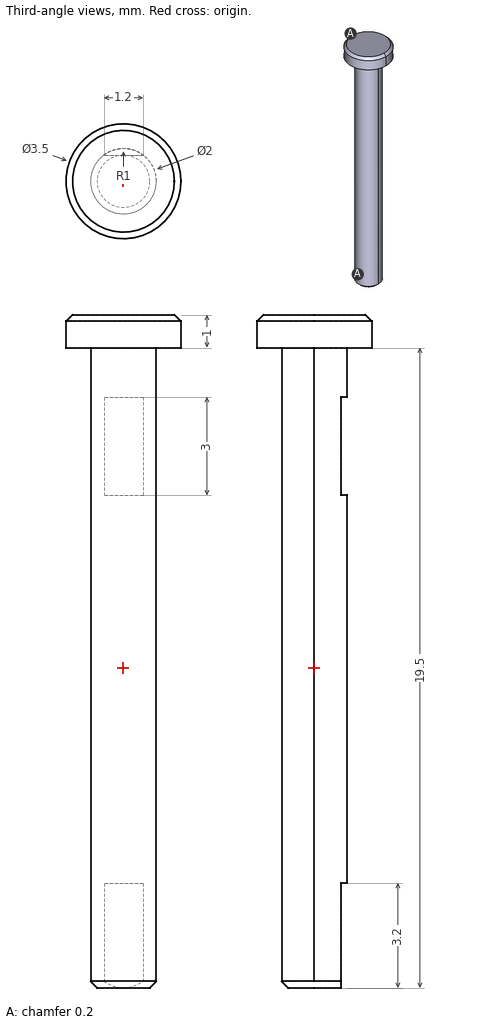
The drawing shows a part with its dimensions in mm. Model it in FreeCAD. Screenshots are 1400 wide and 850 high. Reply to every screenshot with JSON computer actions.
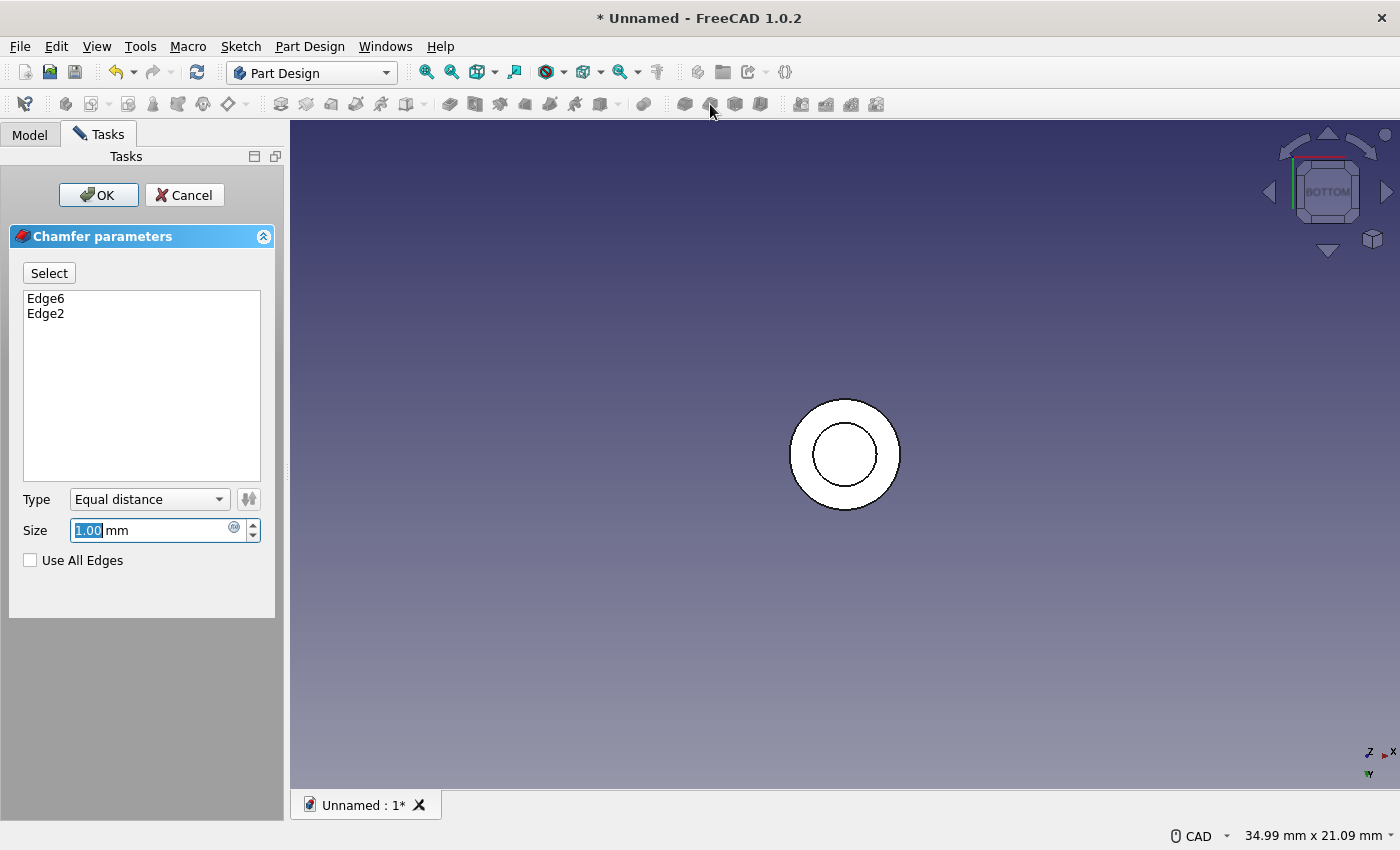
{"action": "type", "text": "0.2"}
{"action": "key", "text": "Tab"}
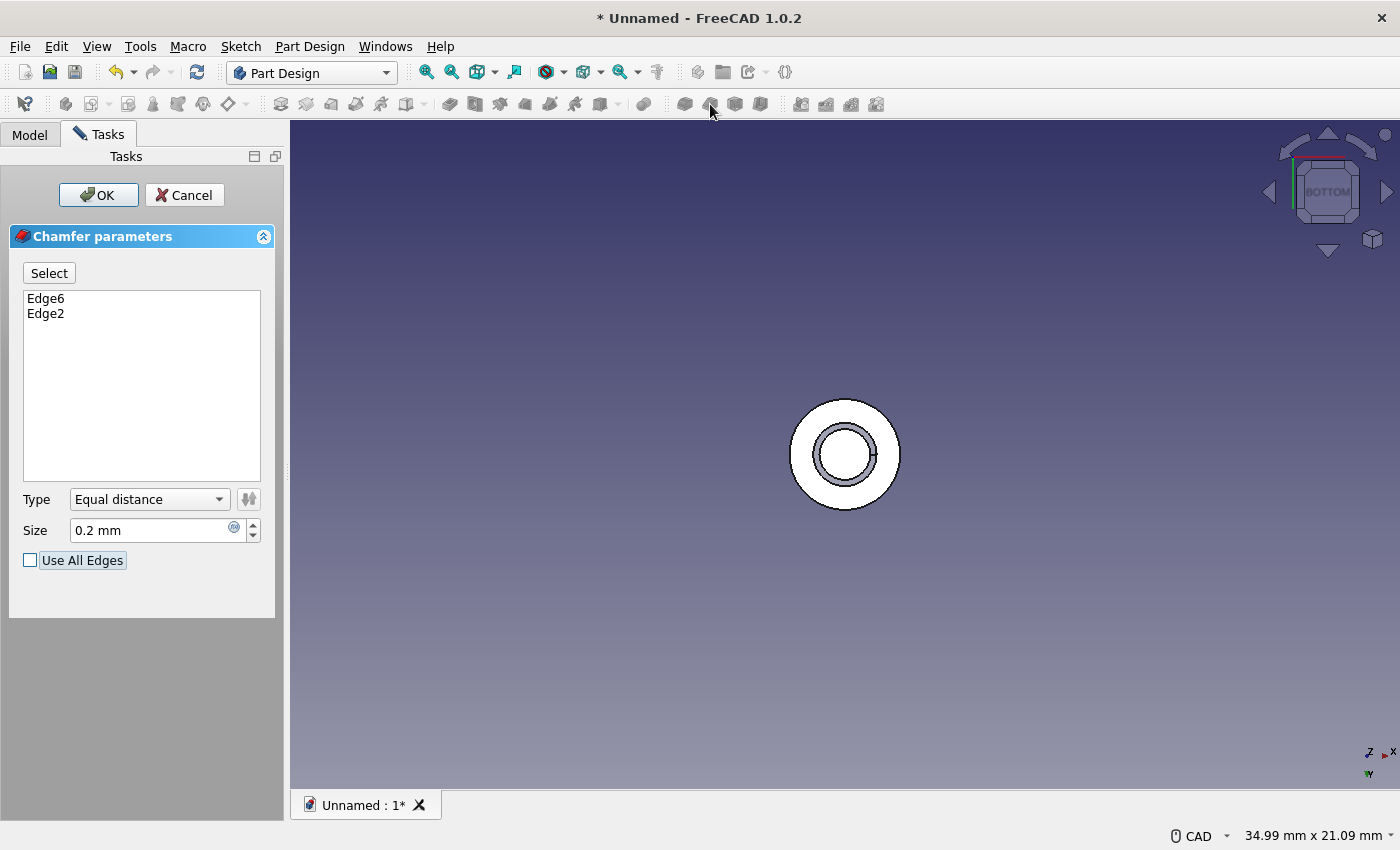
{"action": "left_click", "coordinate": [99, 195]}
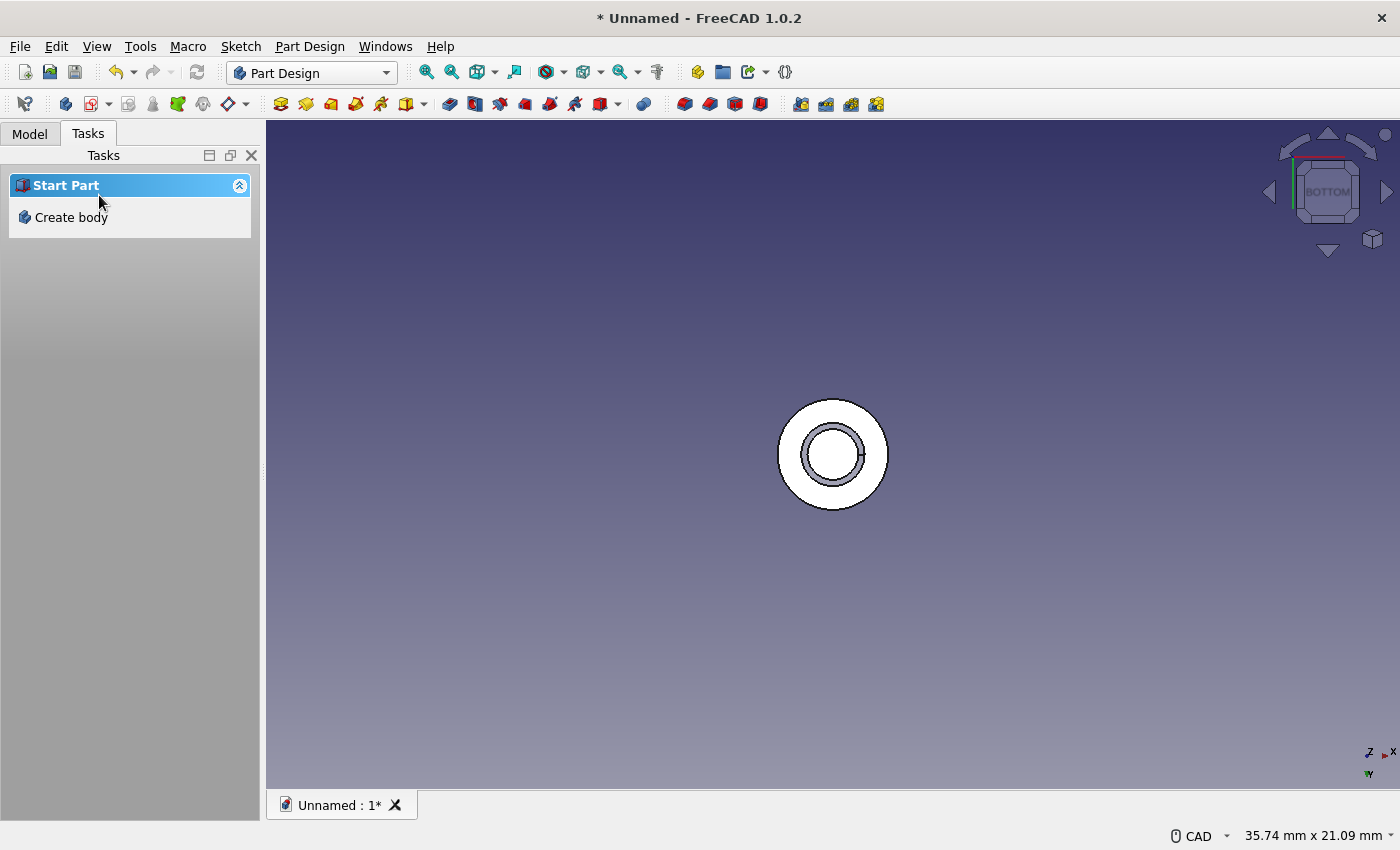
{"action": "left_click", "coordinate": [427, 72]}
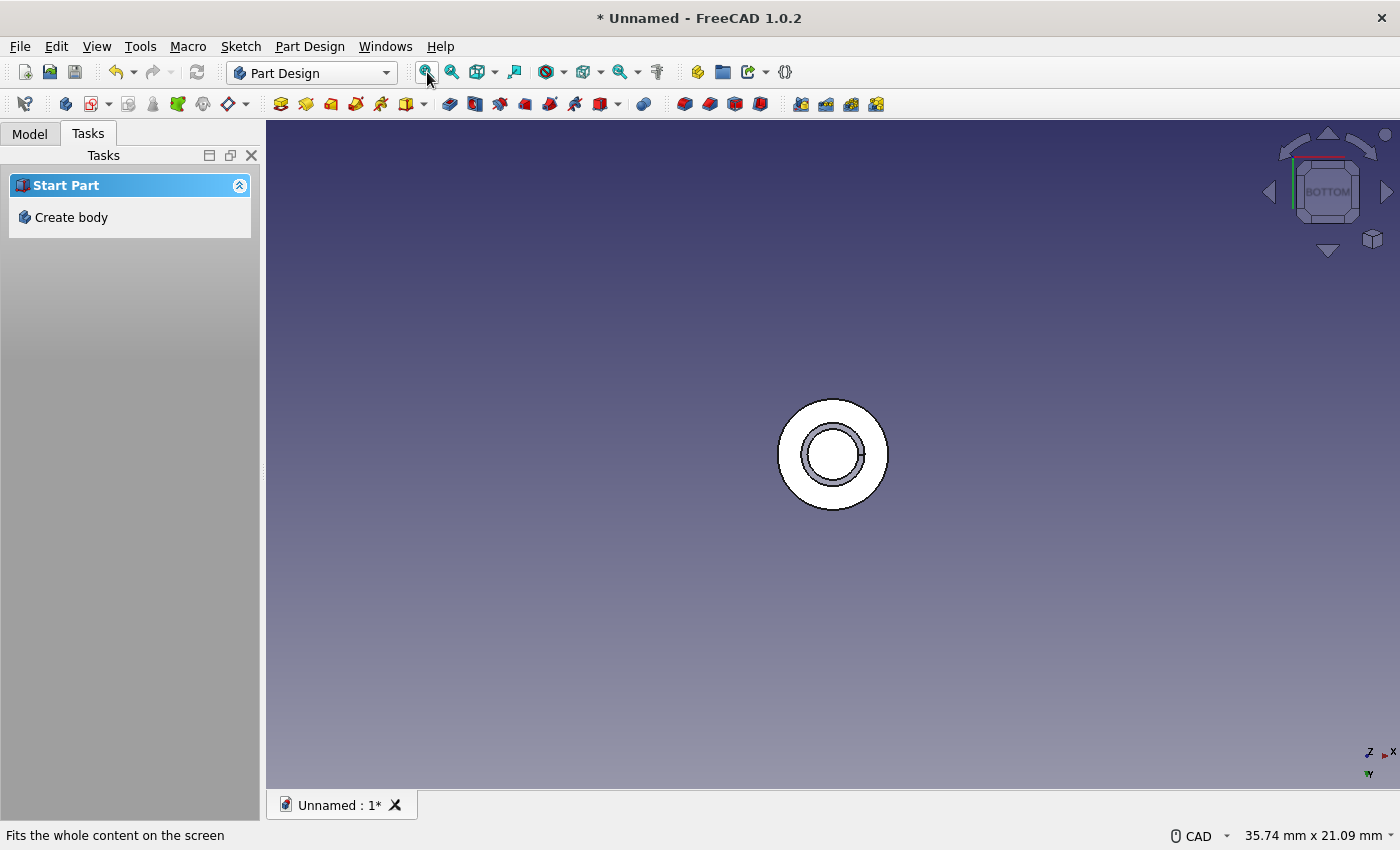
{"action": "left_click", "coordinate": [30, 134]}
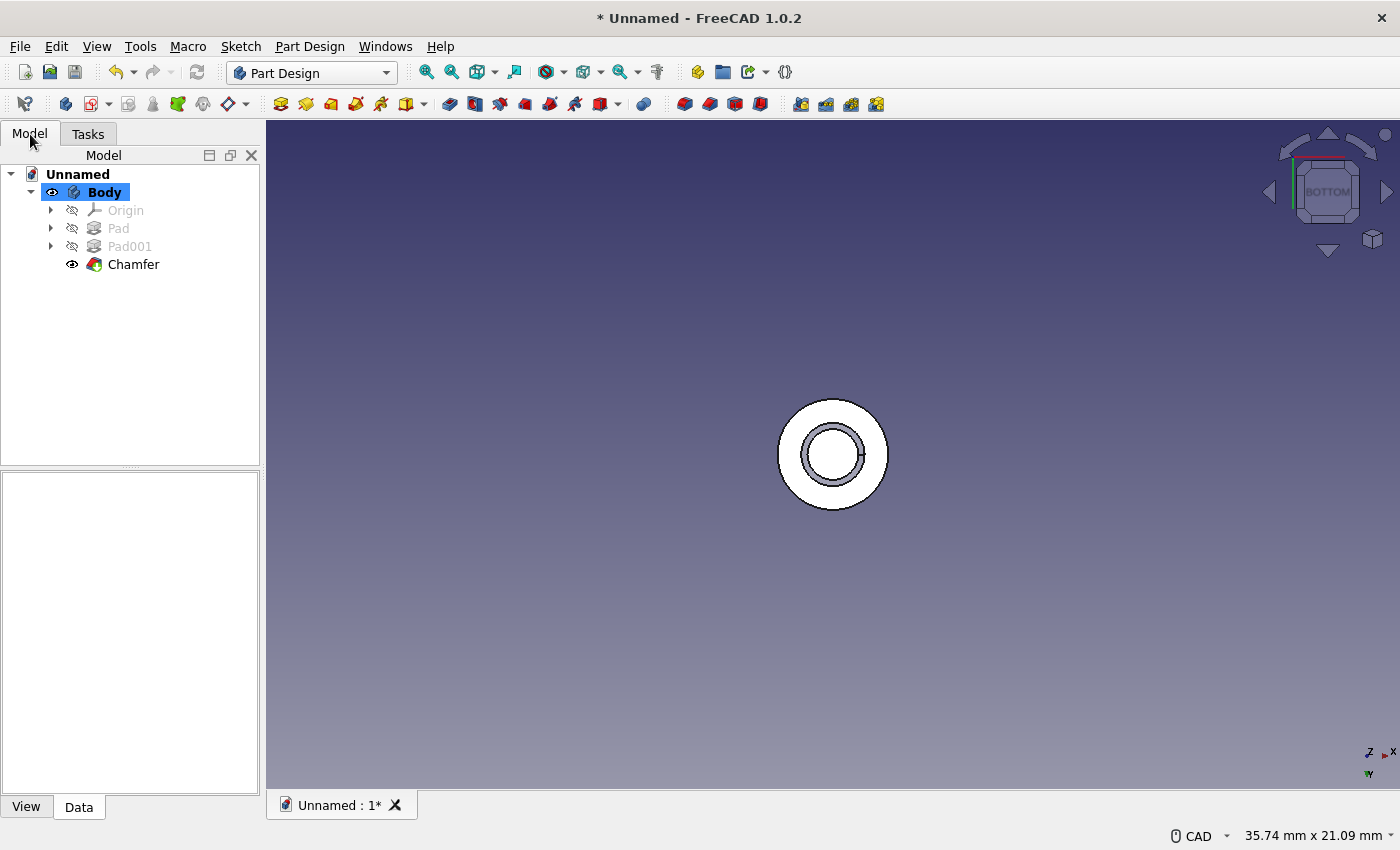
{"action": "left_click", "coordinate": [51, 210]}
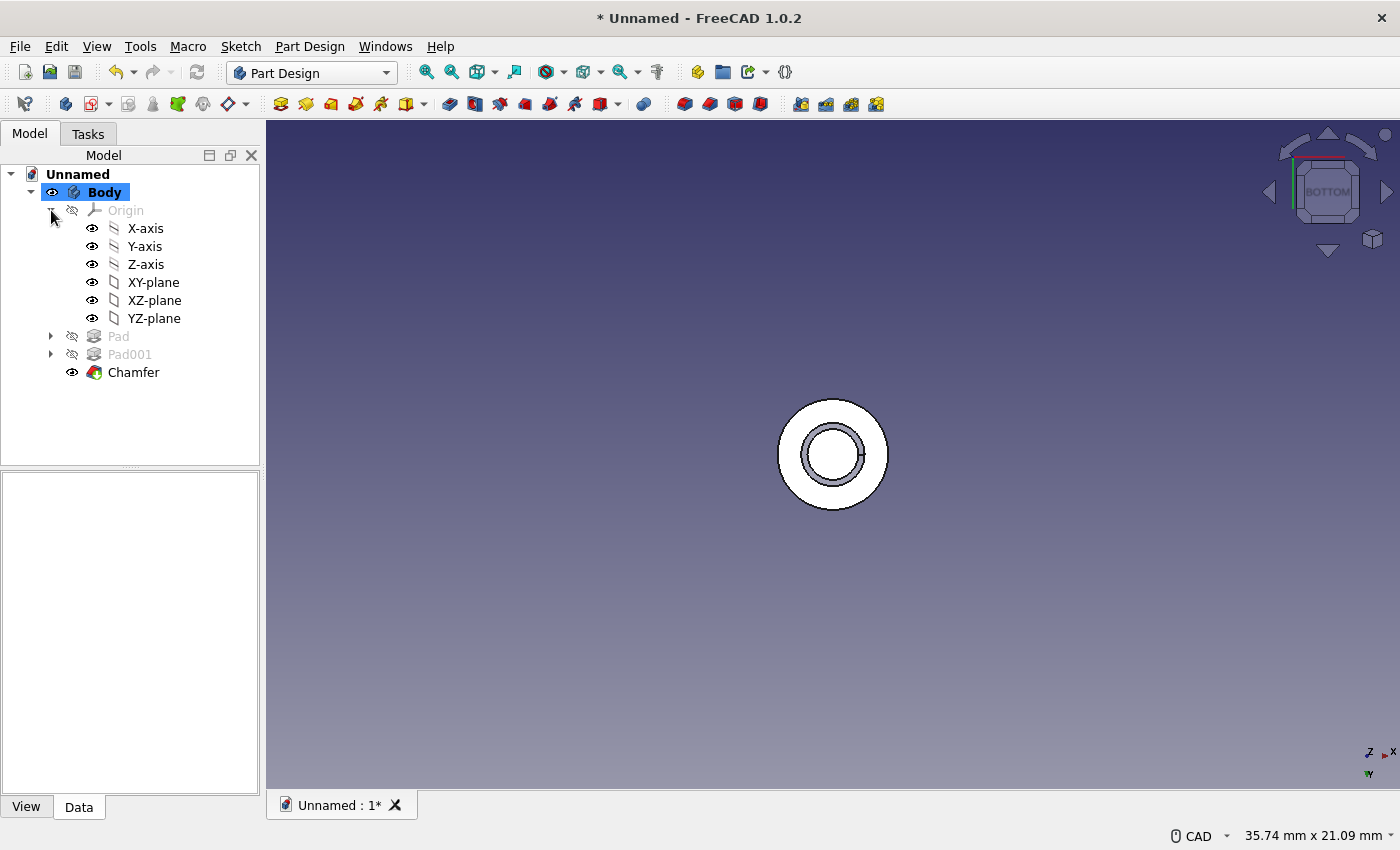
{"action": "left_click", "coordinate": [137, 282]}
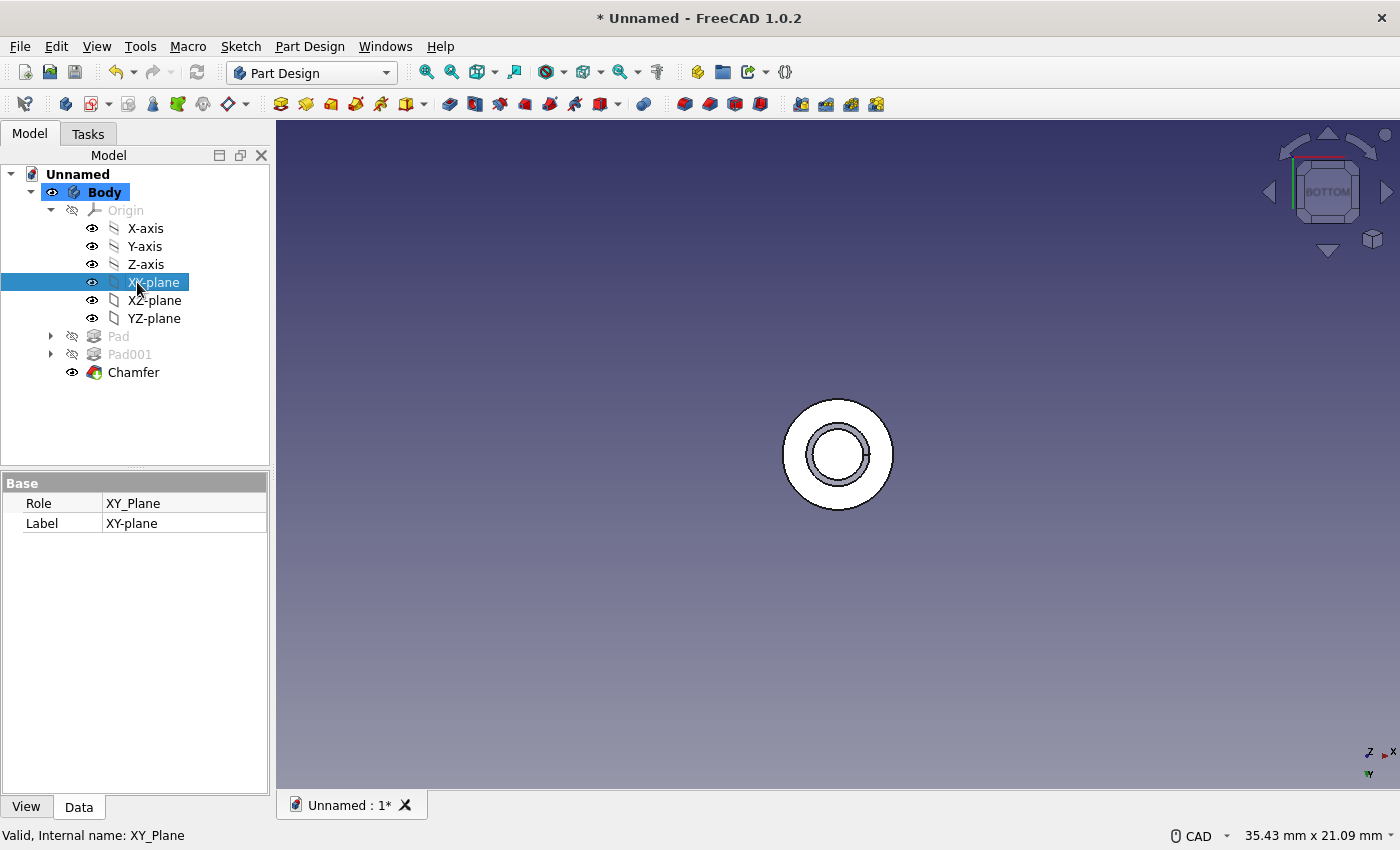
{"action": "left_click", "coordinate": [228, 104]}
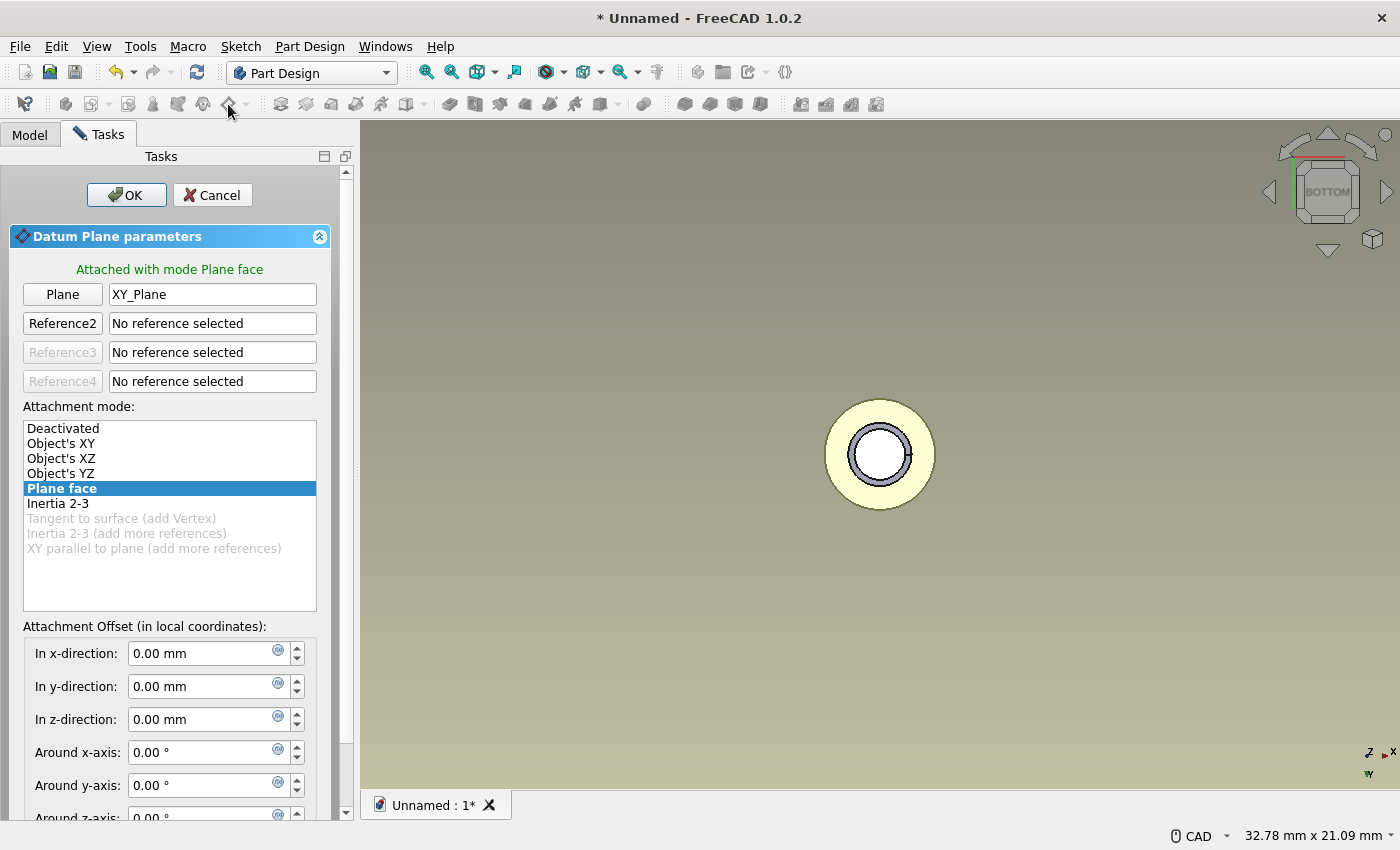
{"action": "triple_click", "coordinate": [210, 720]}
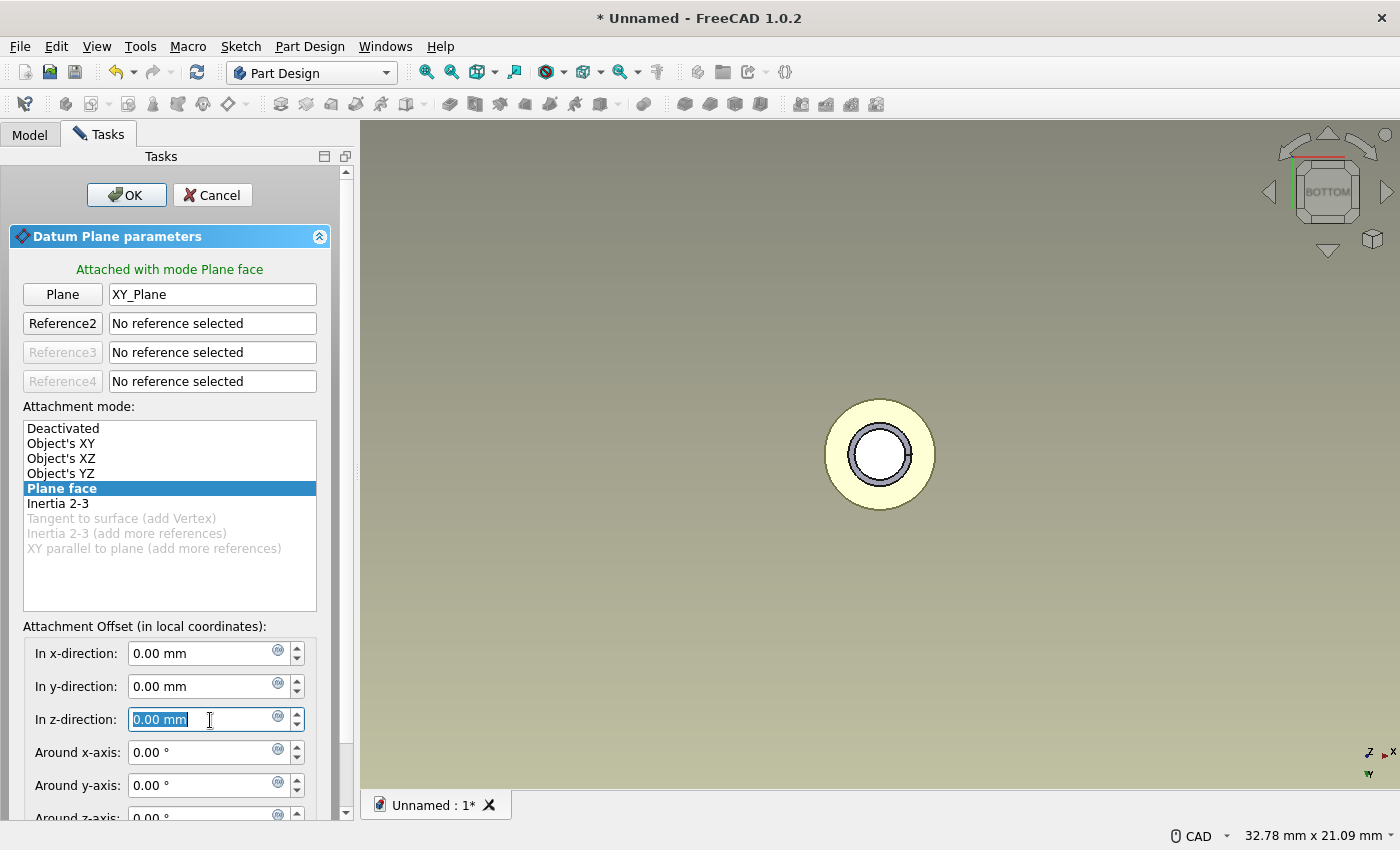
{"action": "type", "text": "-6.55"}
{"action": "key", "text": "Tab"}